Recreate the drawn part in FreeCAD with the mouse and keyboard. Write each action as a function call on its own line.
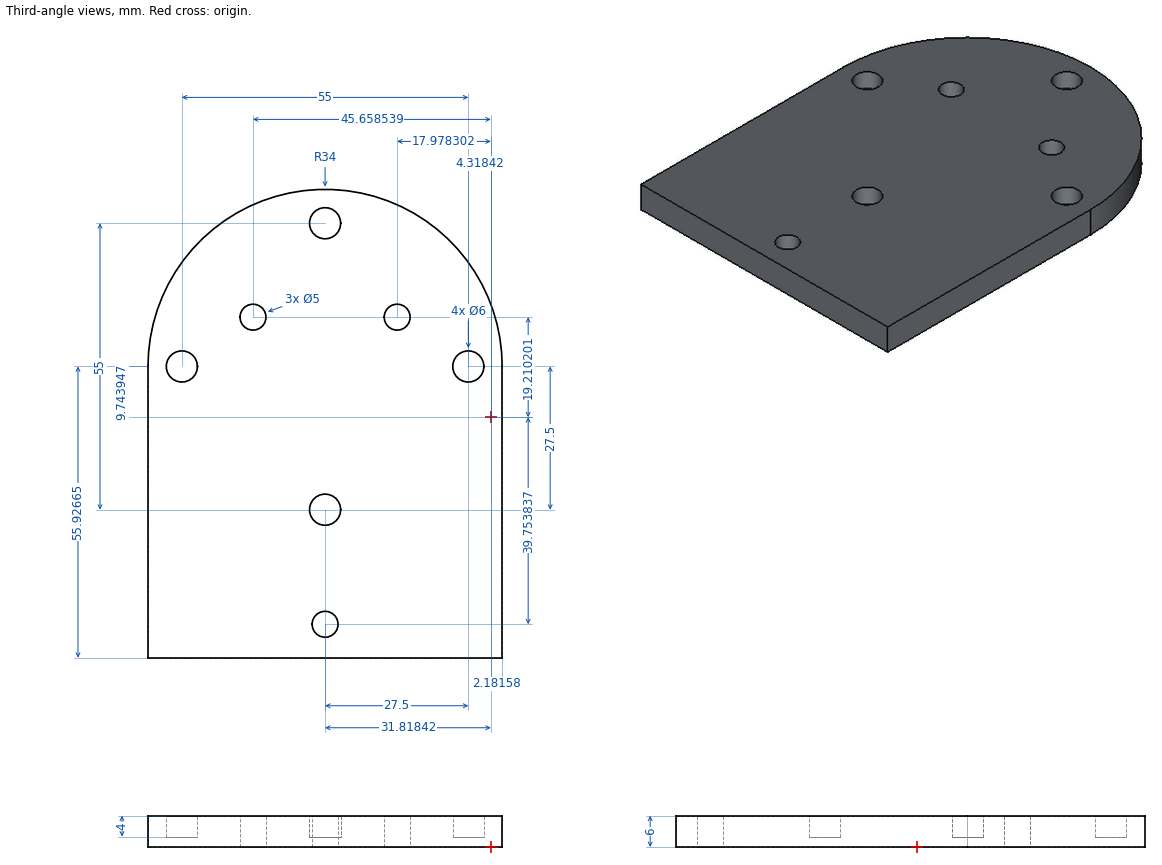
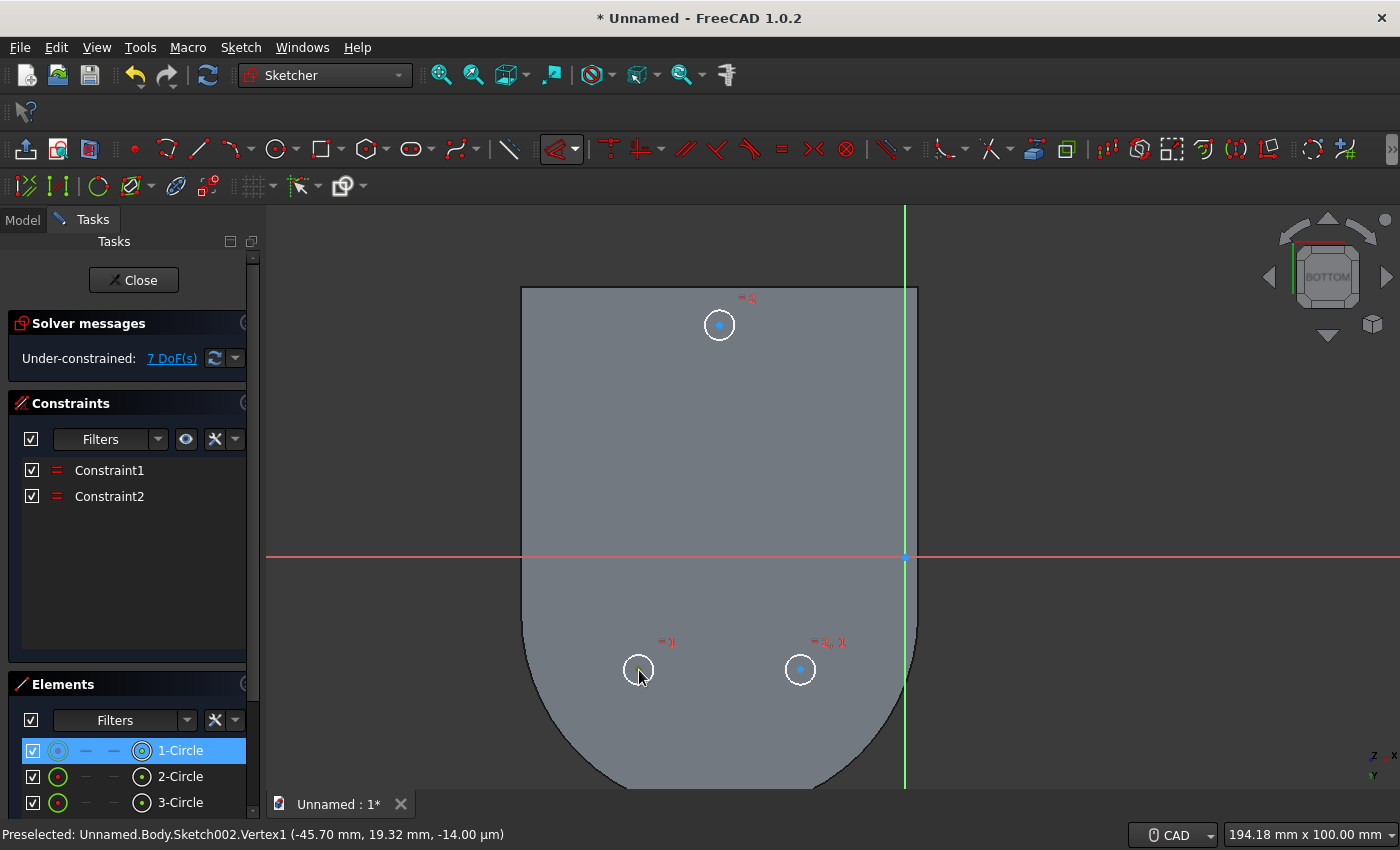
click(800, 670)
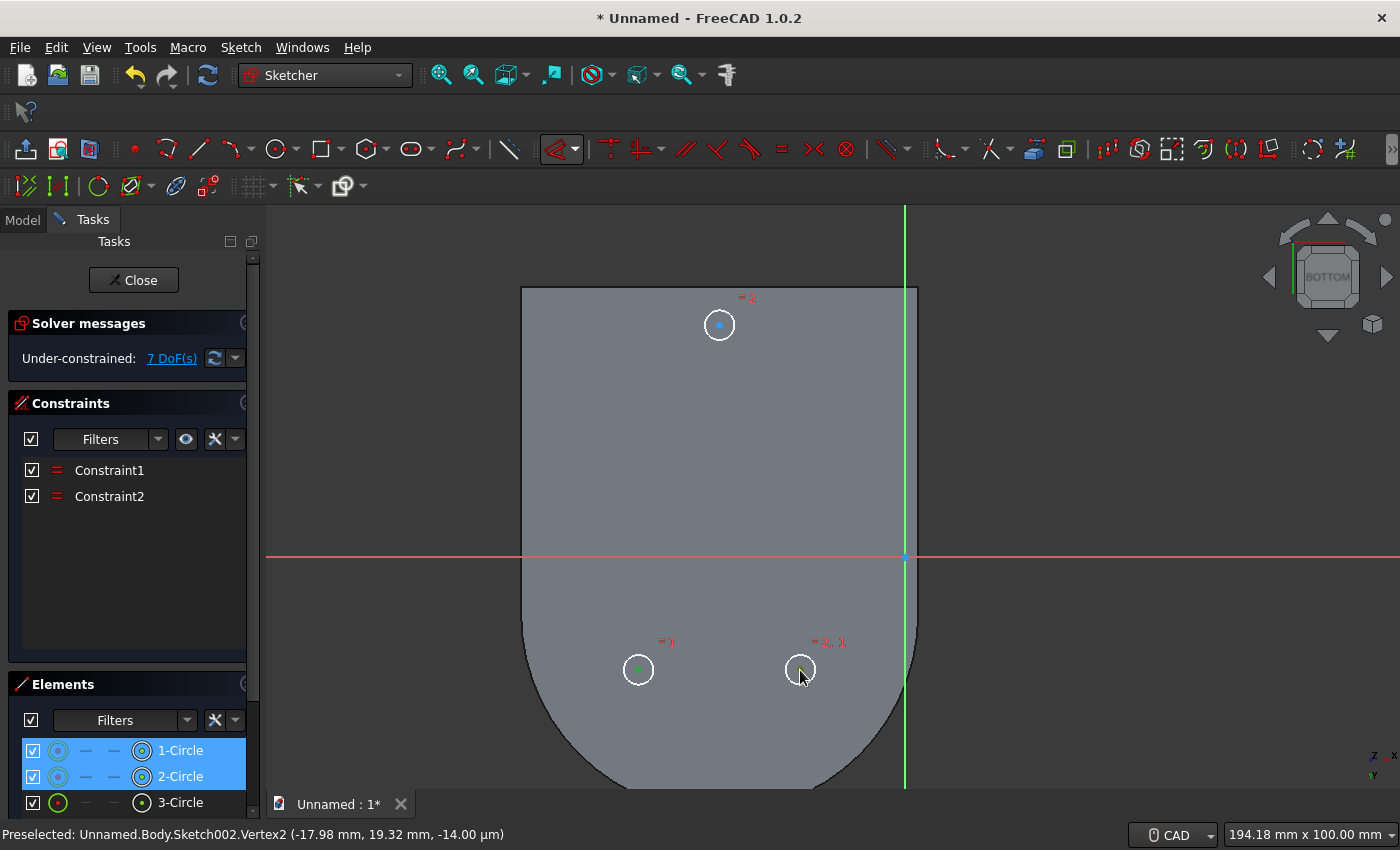
key(h)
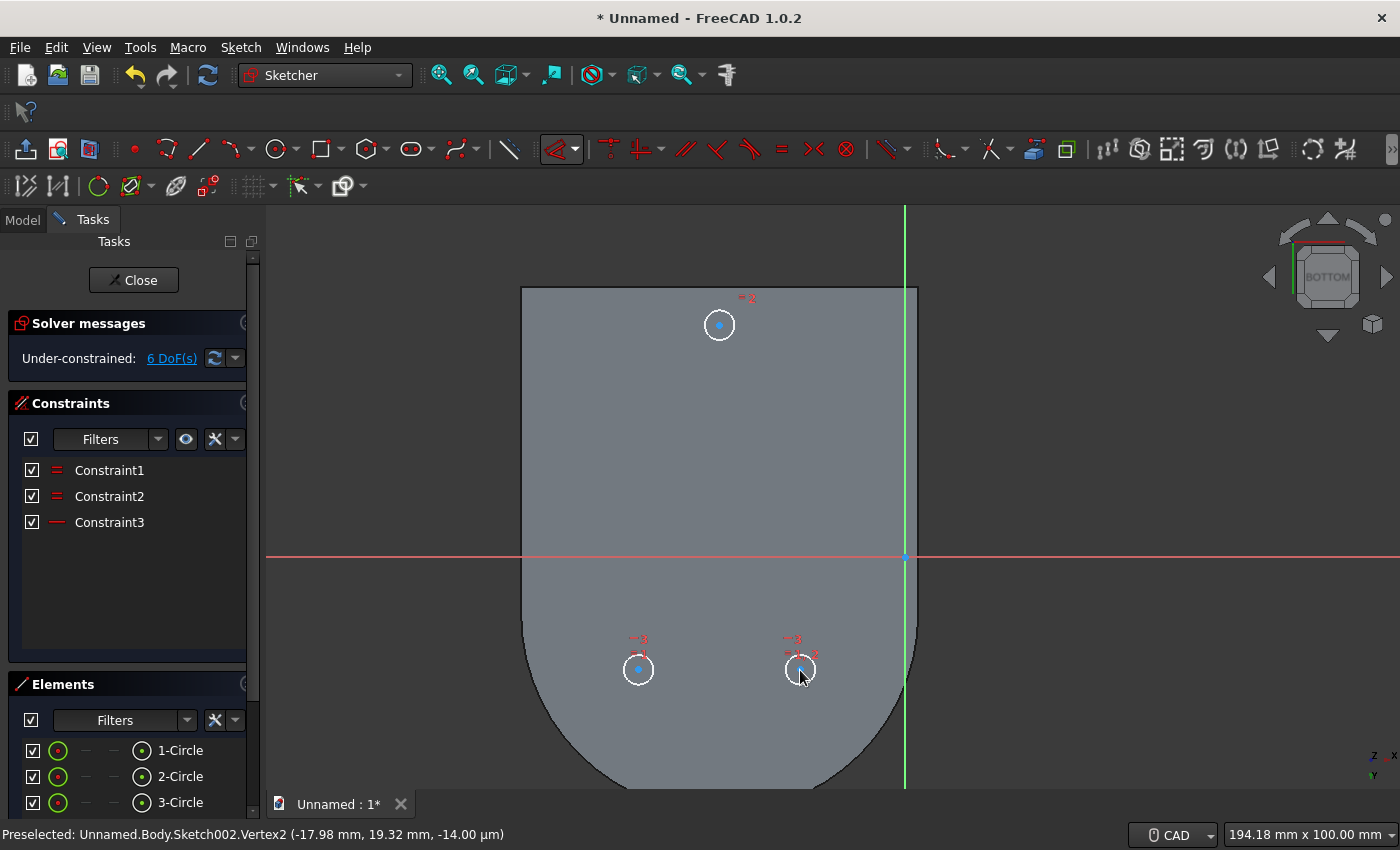
scroll(649, 659, up, 2)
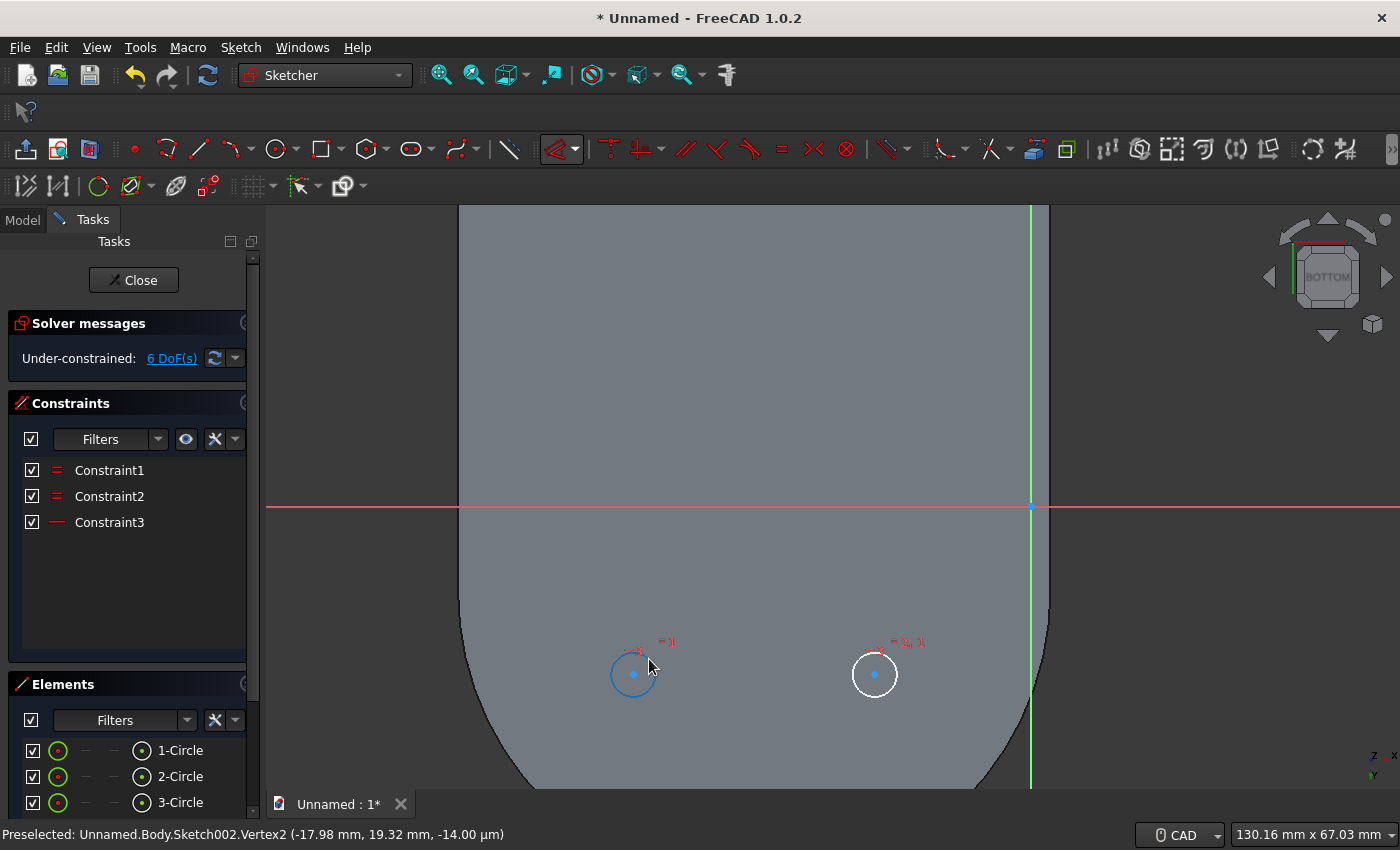
click(649, 659)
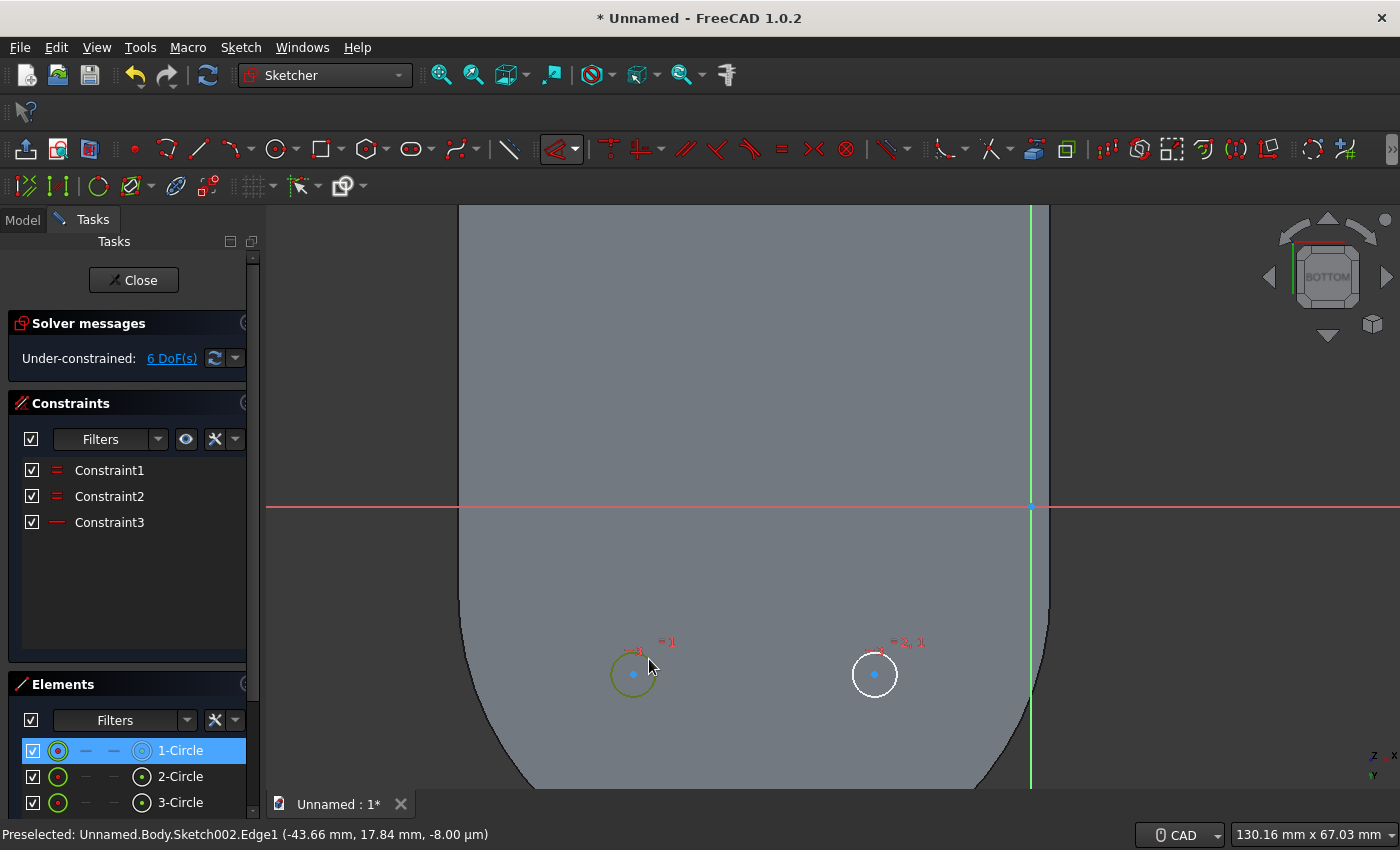
key(k)
key(o)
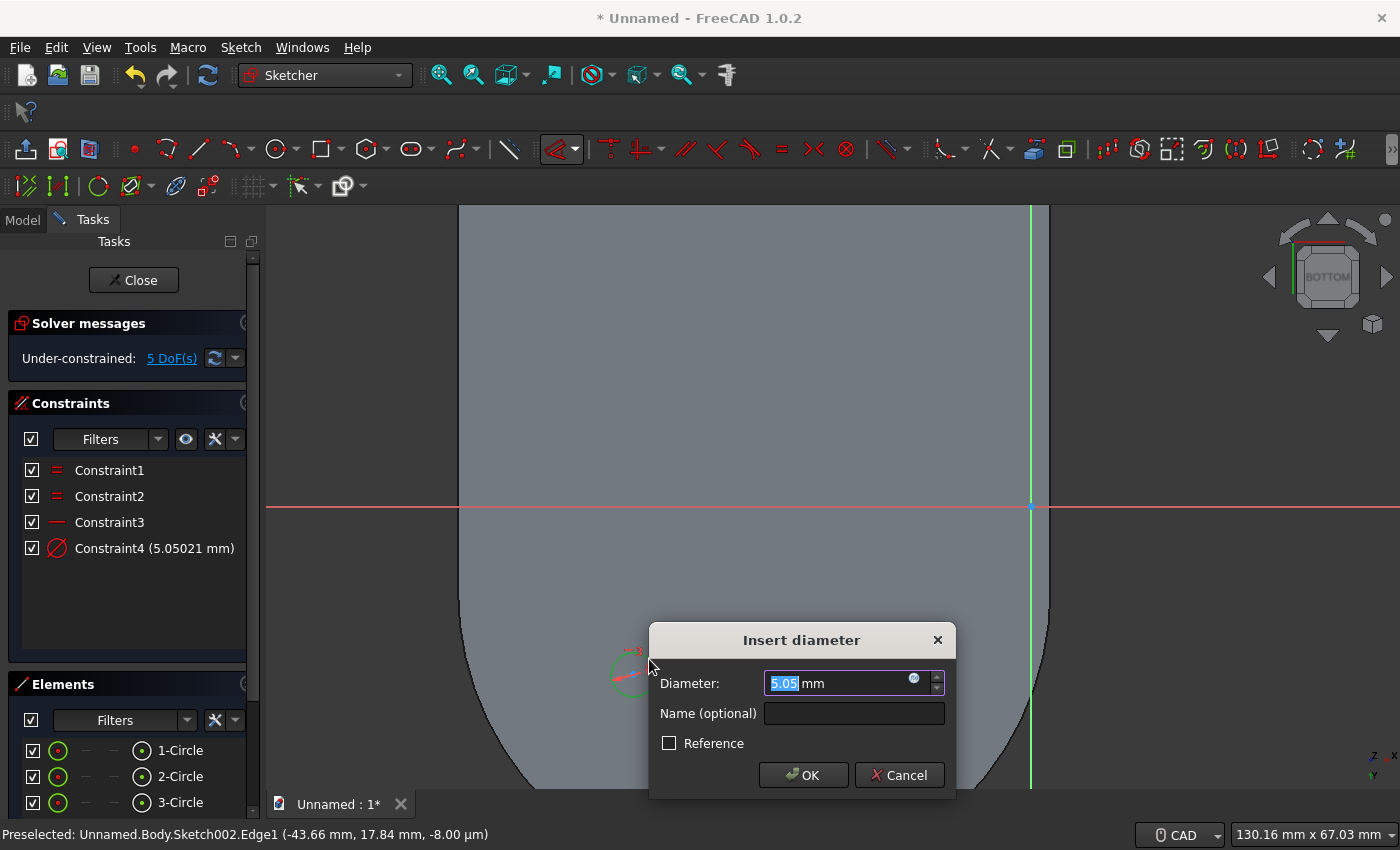
text(5)
key(Return)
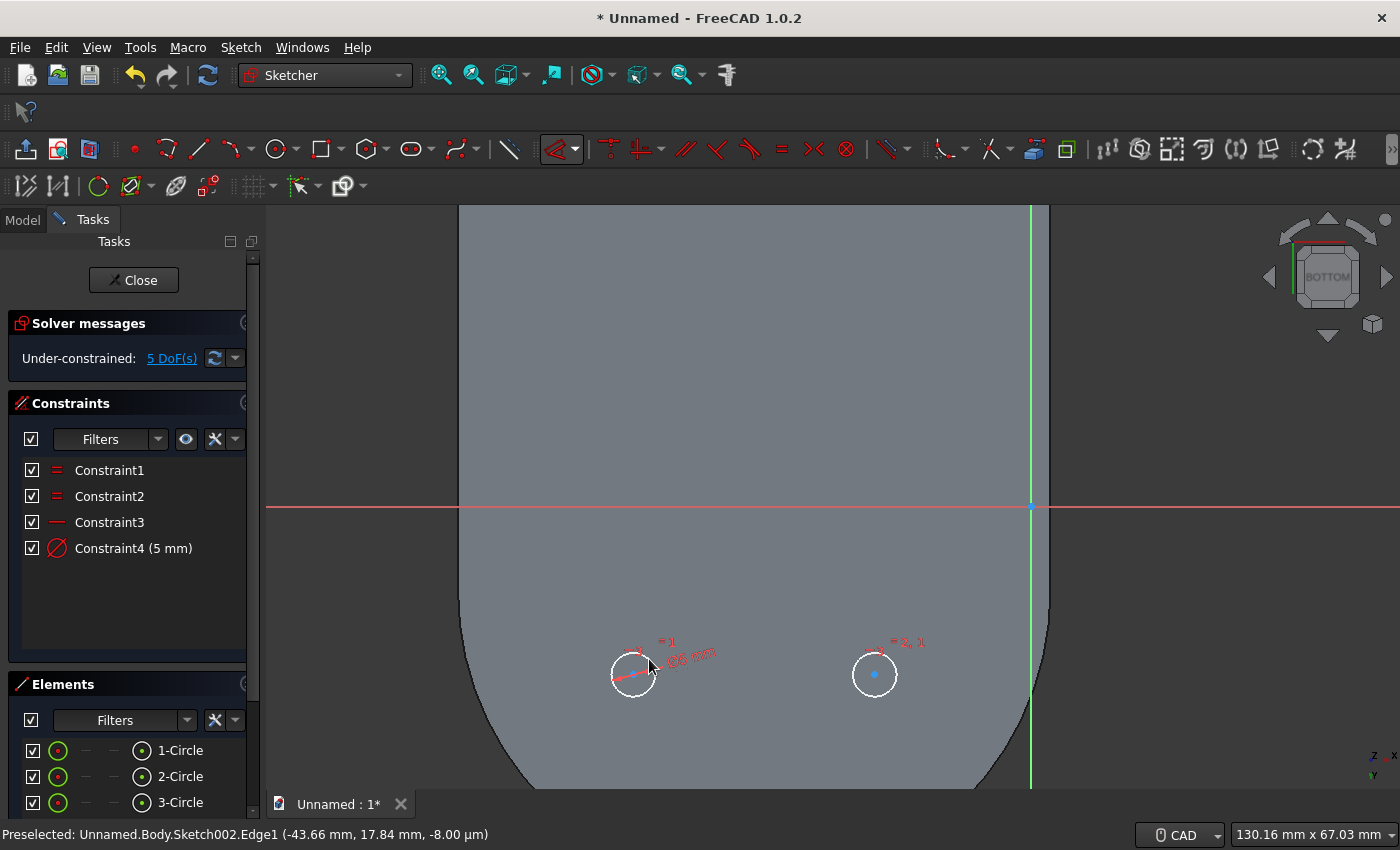
scroll(648, 660, down, 2)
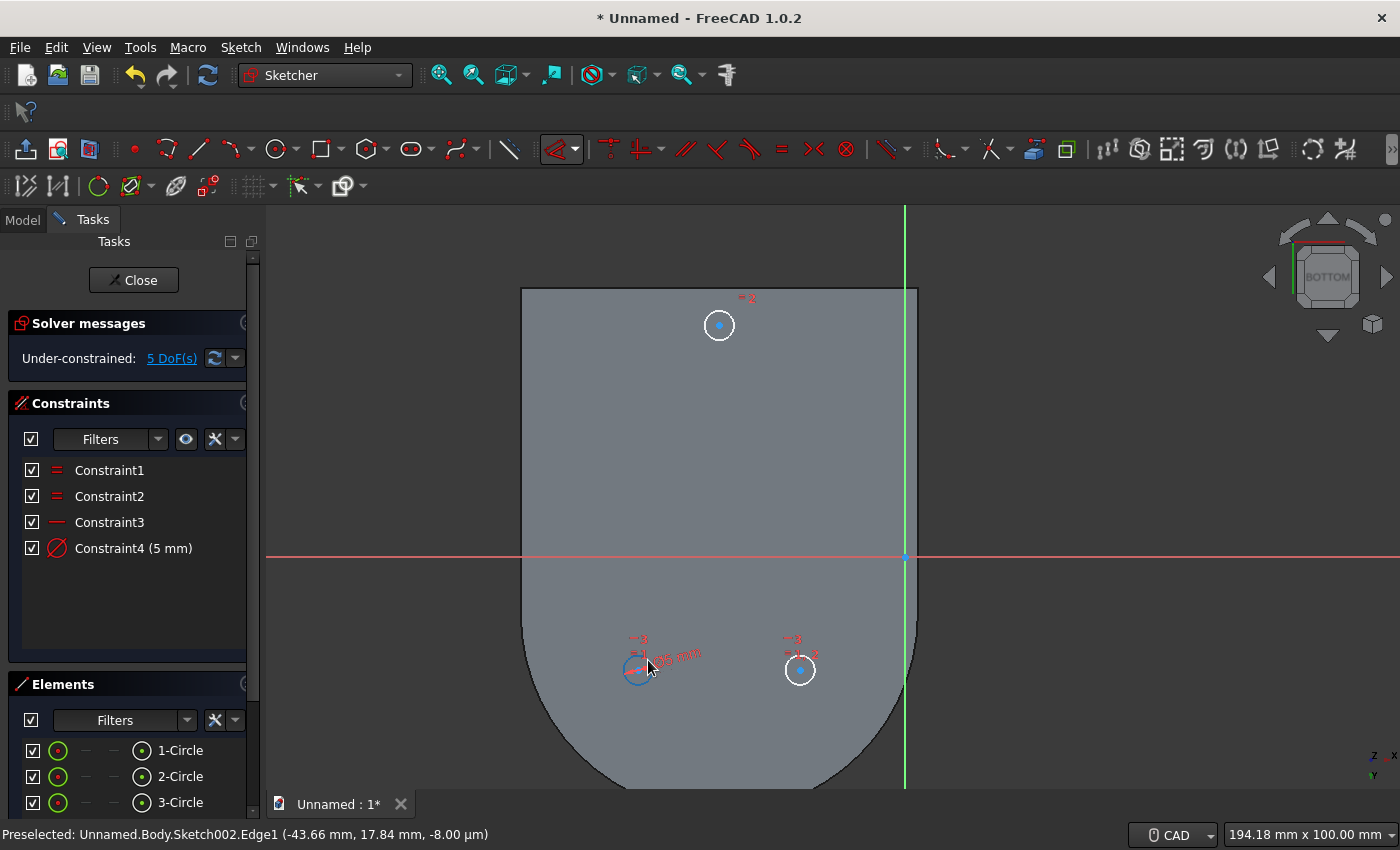
click(719, 326)